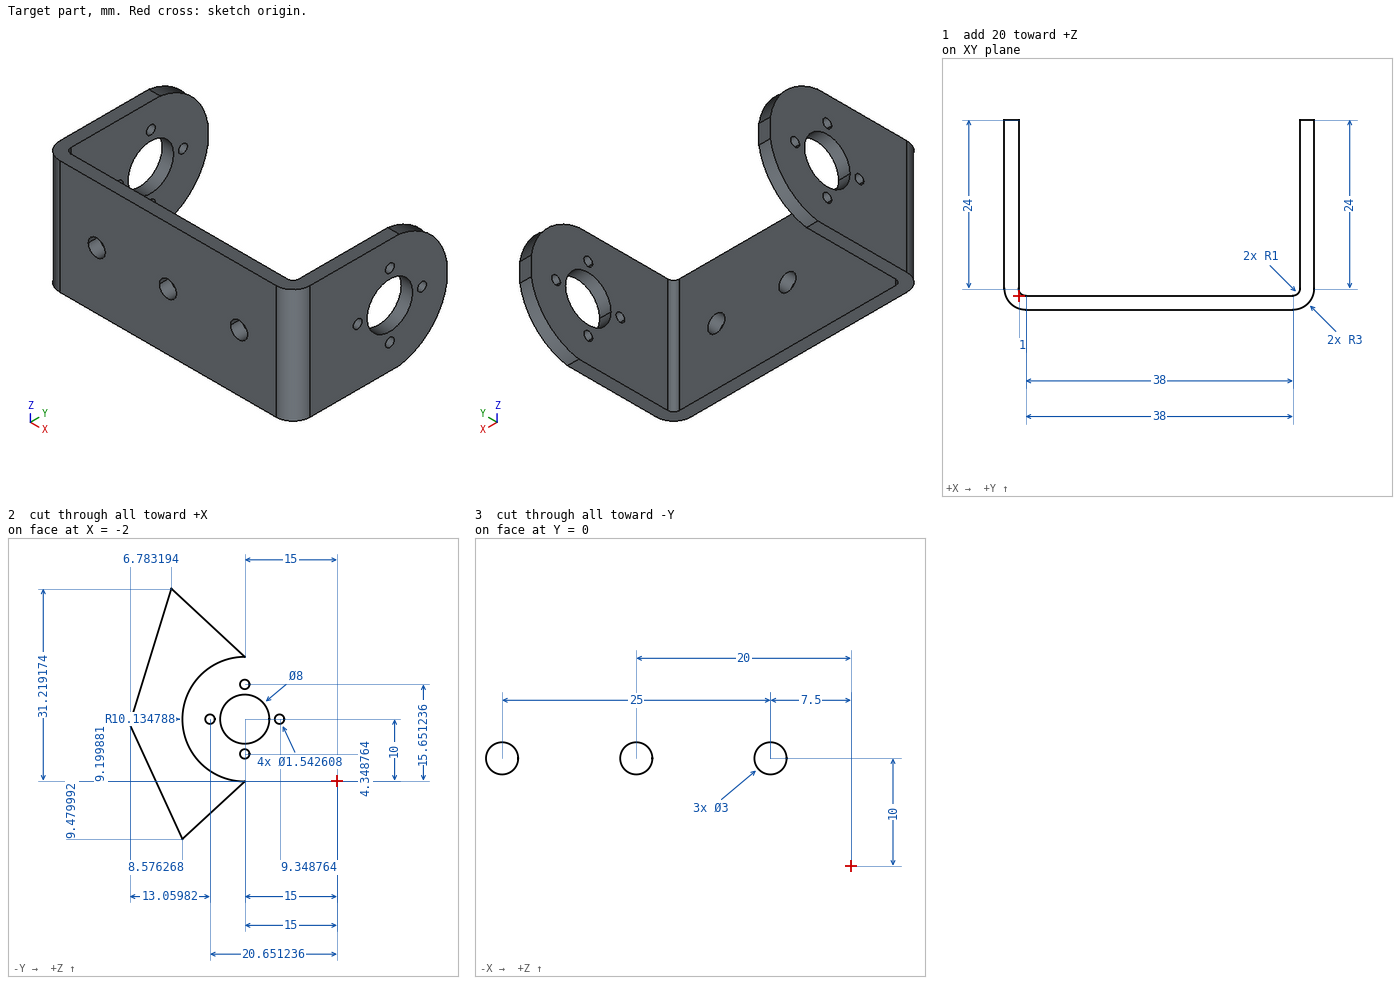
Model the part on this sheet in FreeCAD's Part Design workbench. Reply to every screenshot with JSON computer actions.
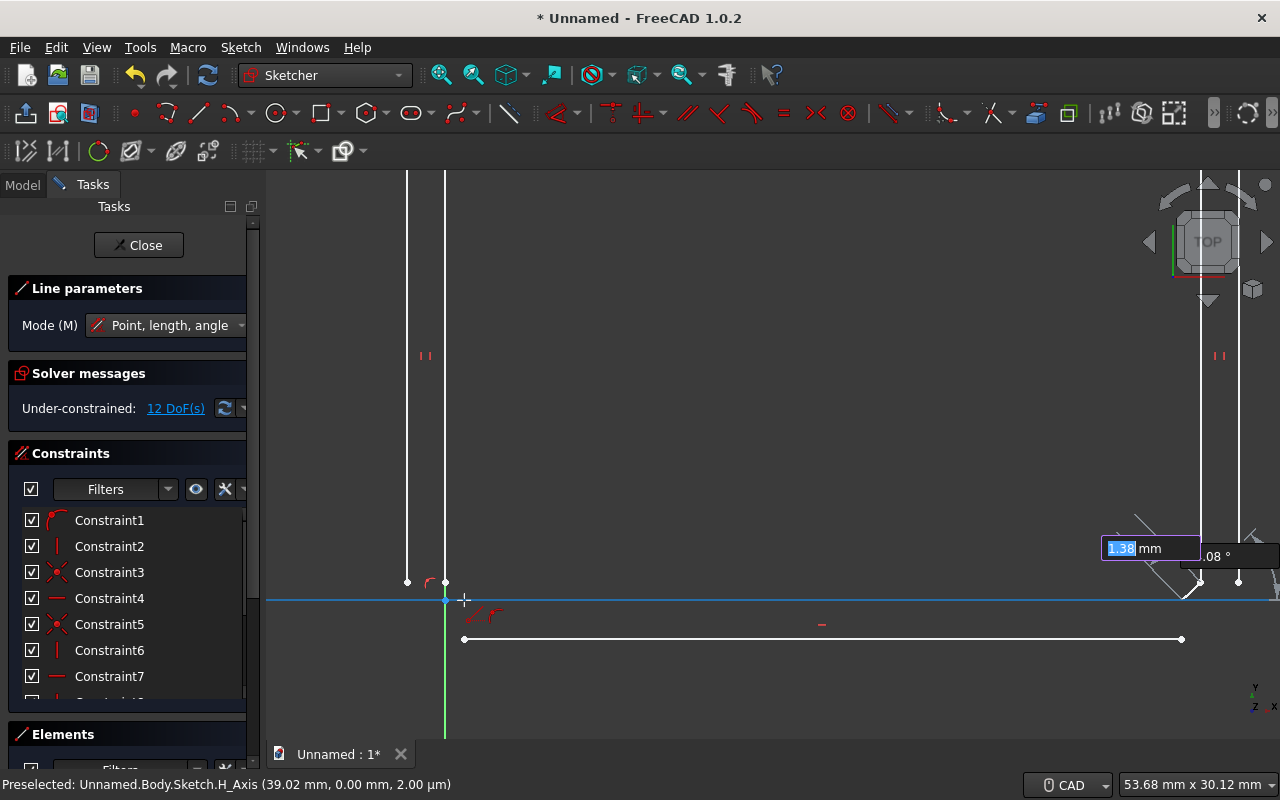
{"action": "left_click", "coordinate": [464, 591]}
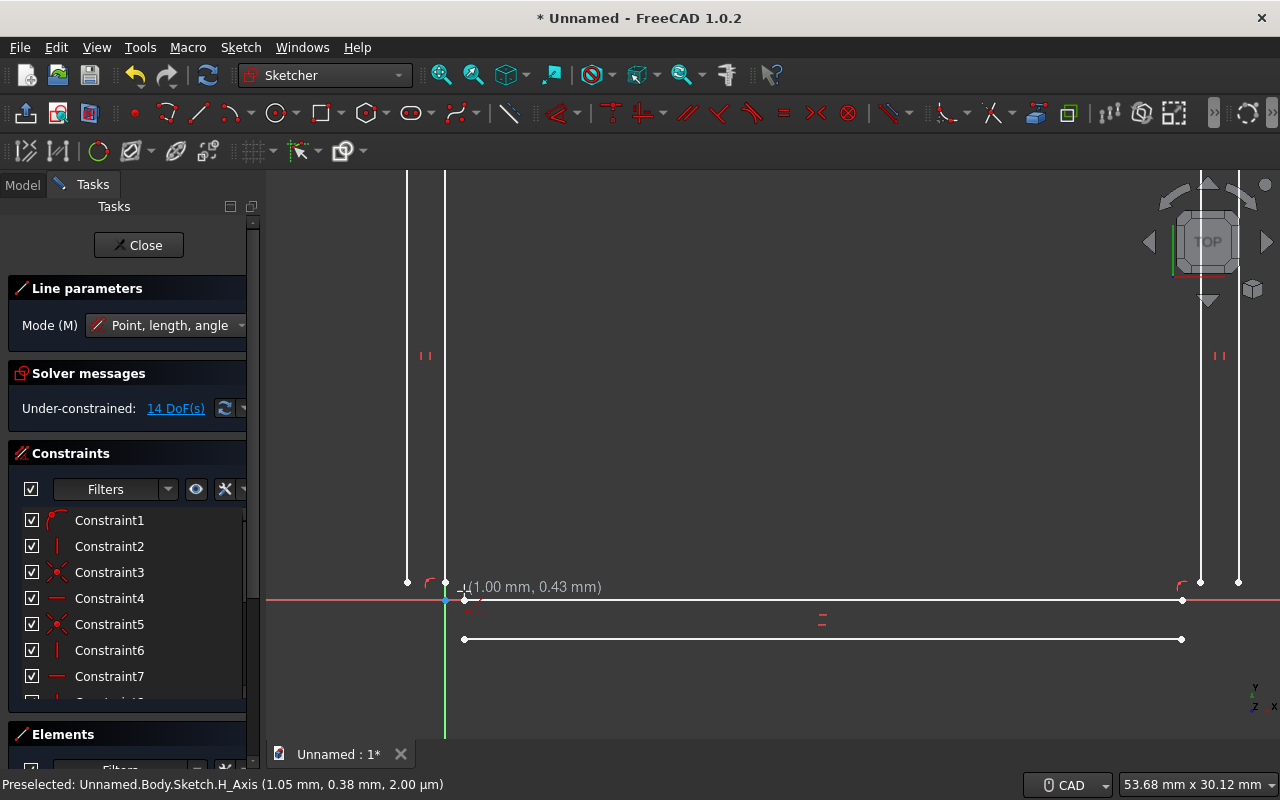
{"action": "left_click", "coordinate": [254, 114]}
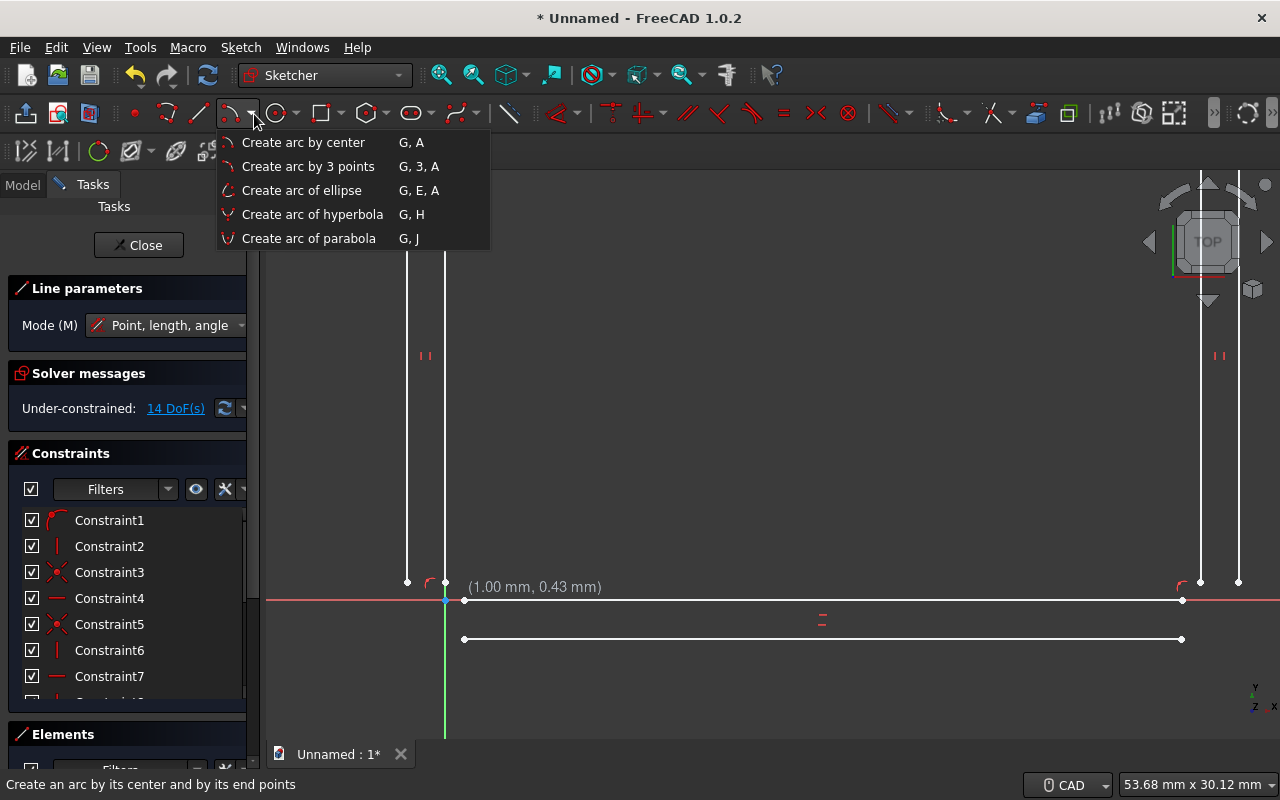
{"action": "left_click", "coordinate": [354, 166]}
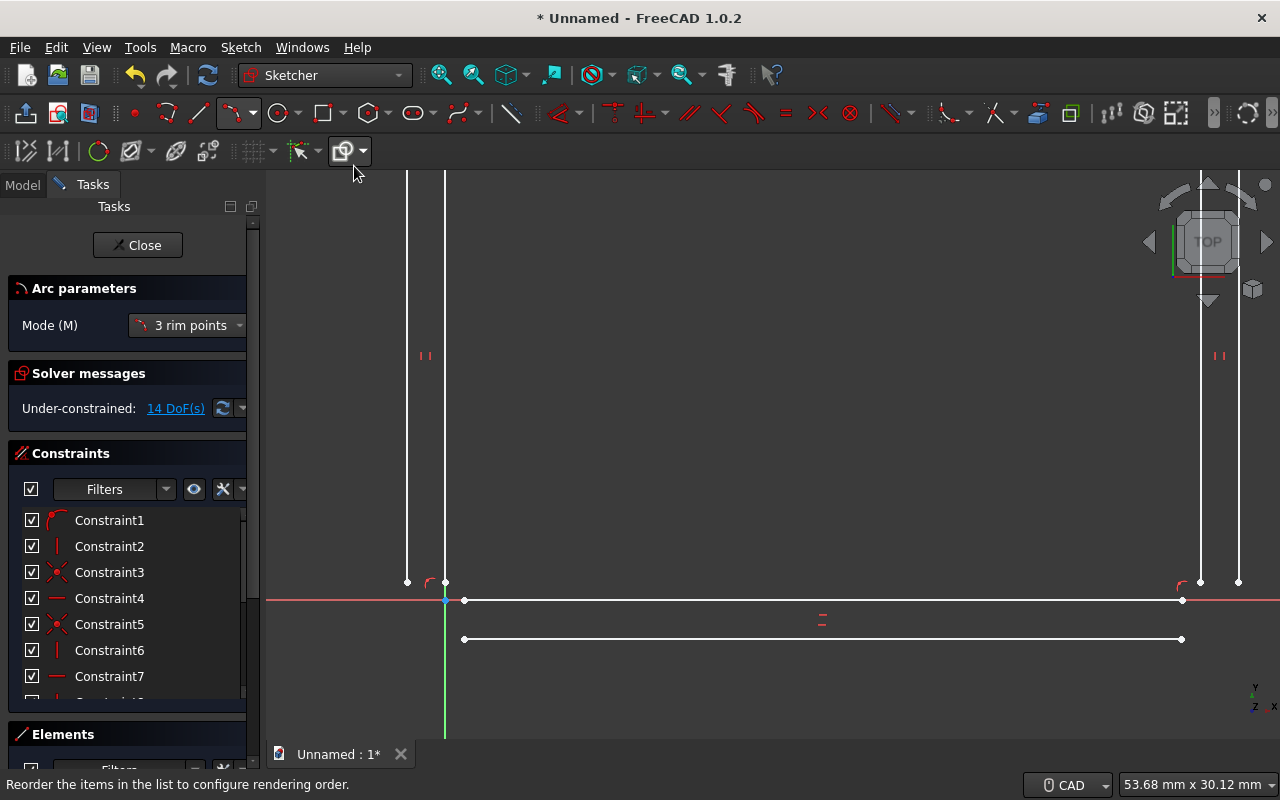
{"action": "left_click", "coordinate": [407, 582]}
{"action": "left_click", "coordinate": [464, 639]}
{"action": "left_click", "coordinate": [424, 621]}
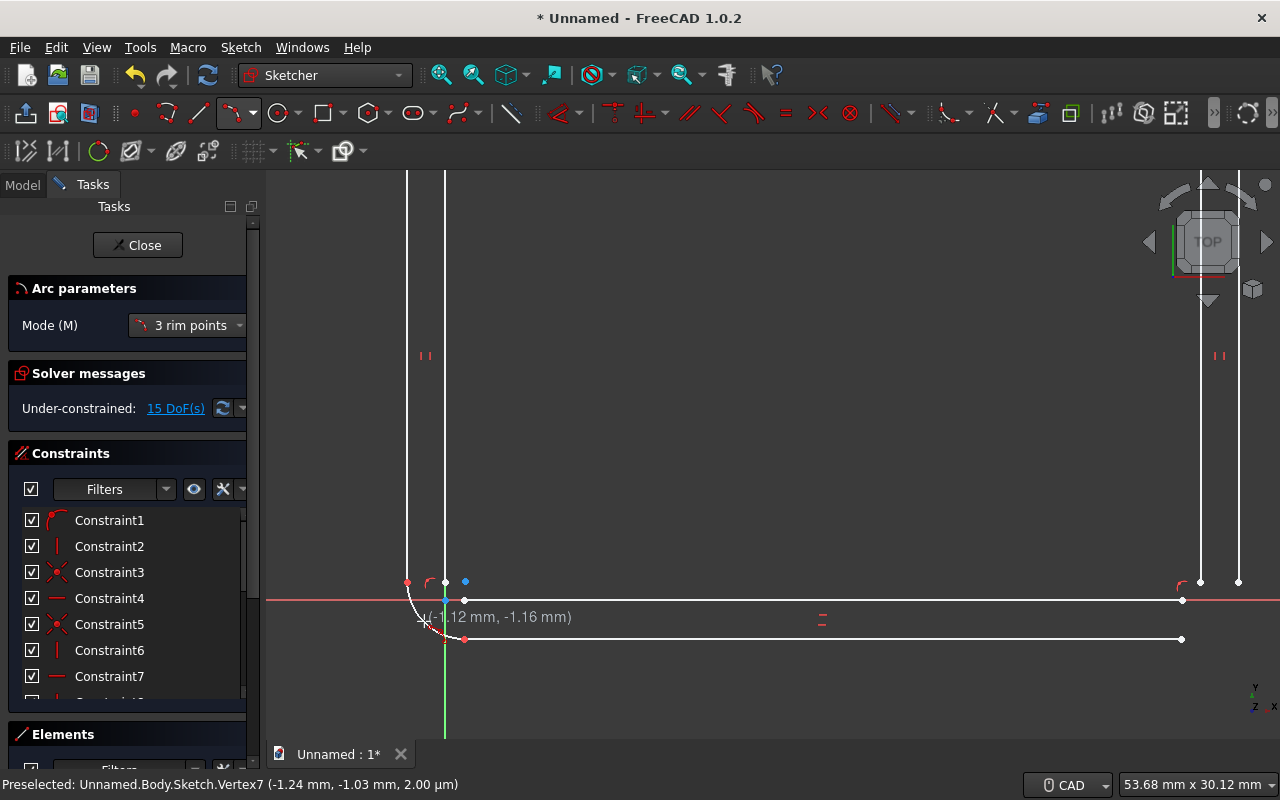
{"action": "scroll", "coordinate": [464, 600], "scroll_direction": "down", "scroll_amount": 2}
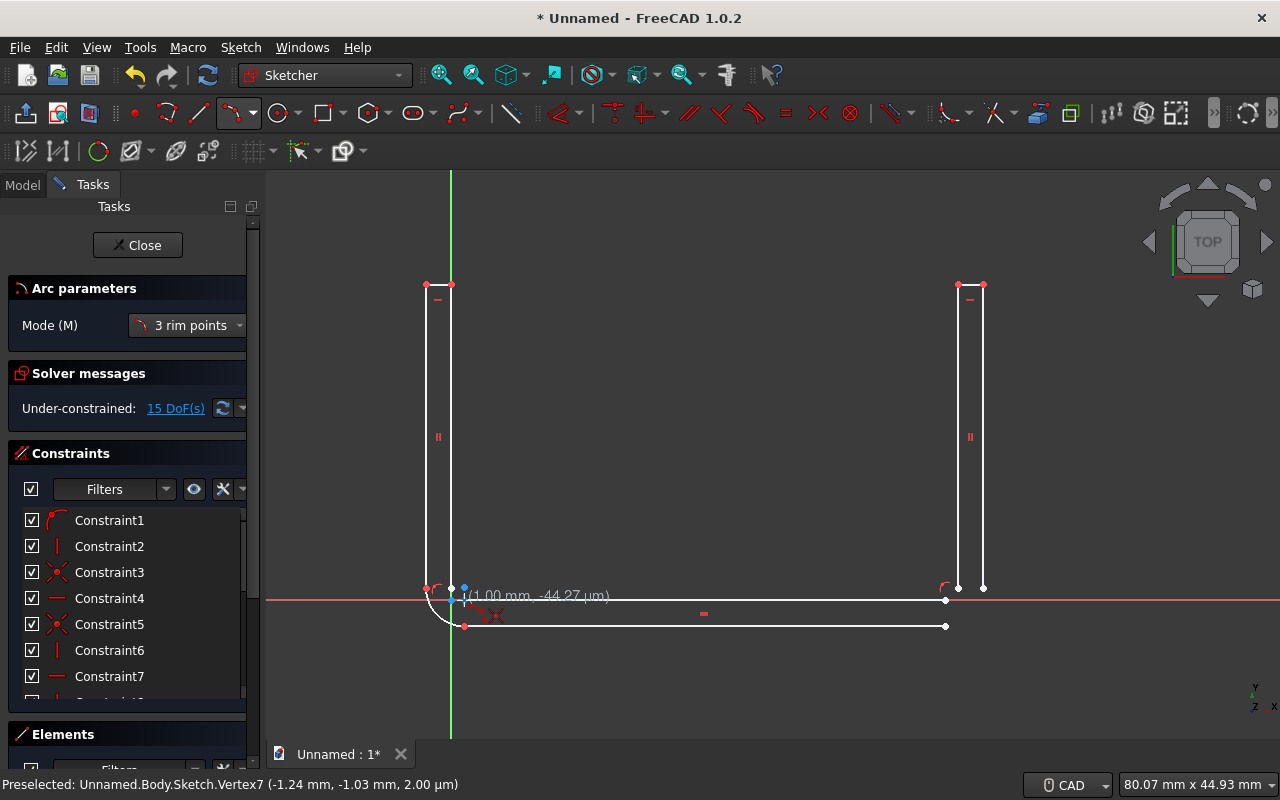
{"action": "left_click", "coordinate": [945, 626]}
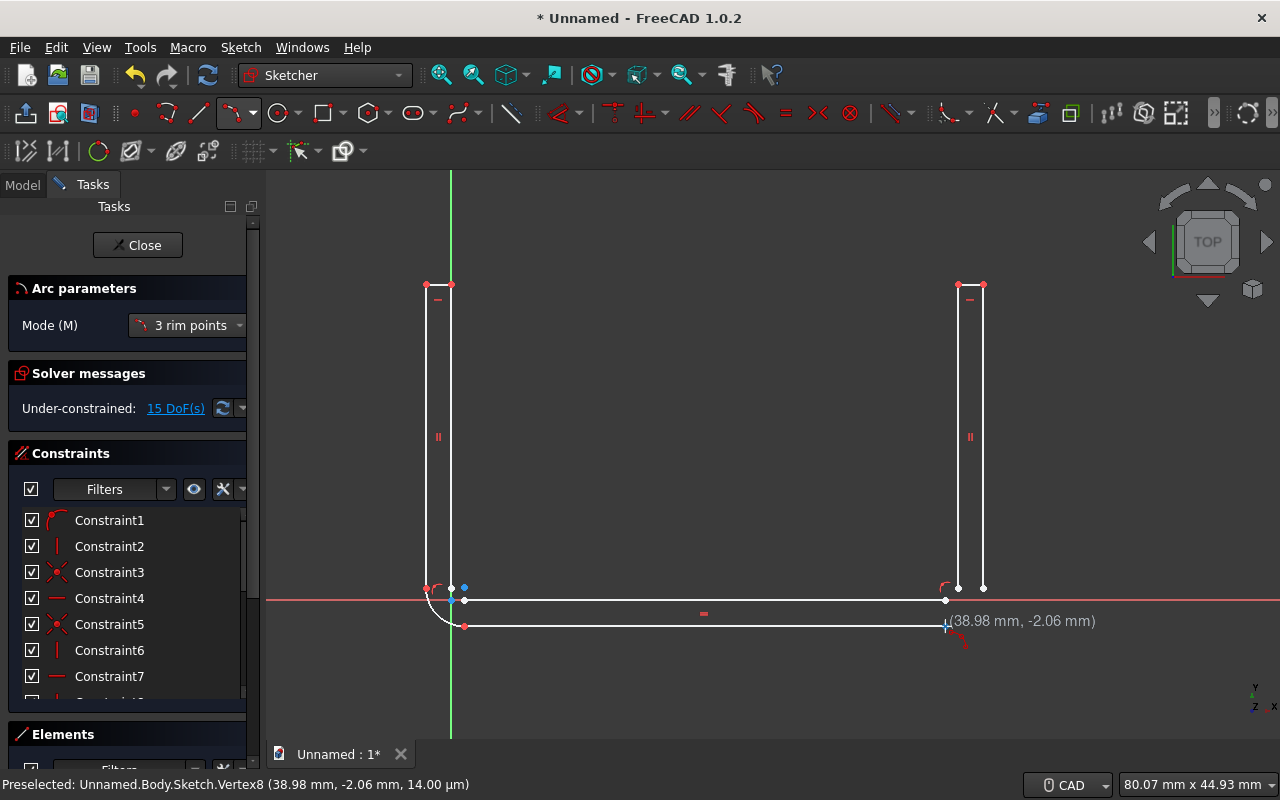
{"action": "scroll", "coordinate": [983, 588], "scroll_direction": "up", "scroll_amount": 2}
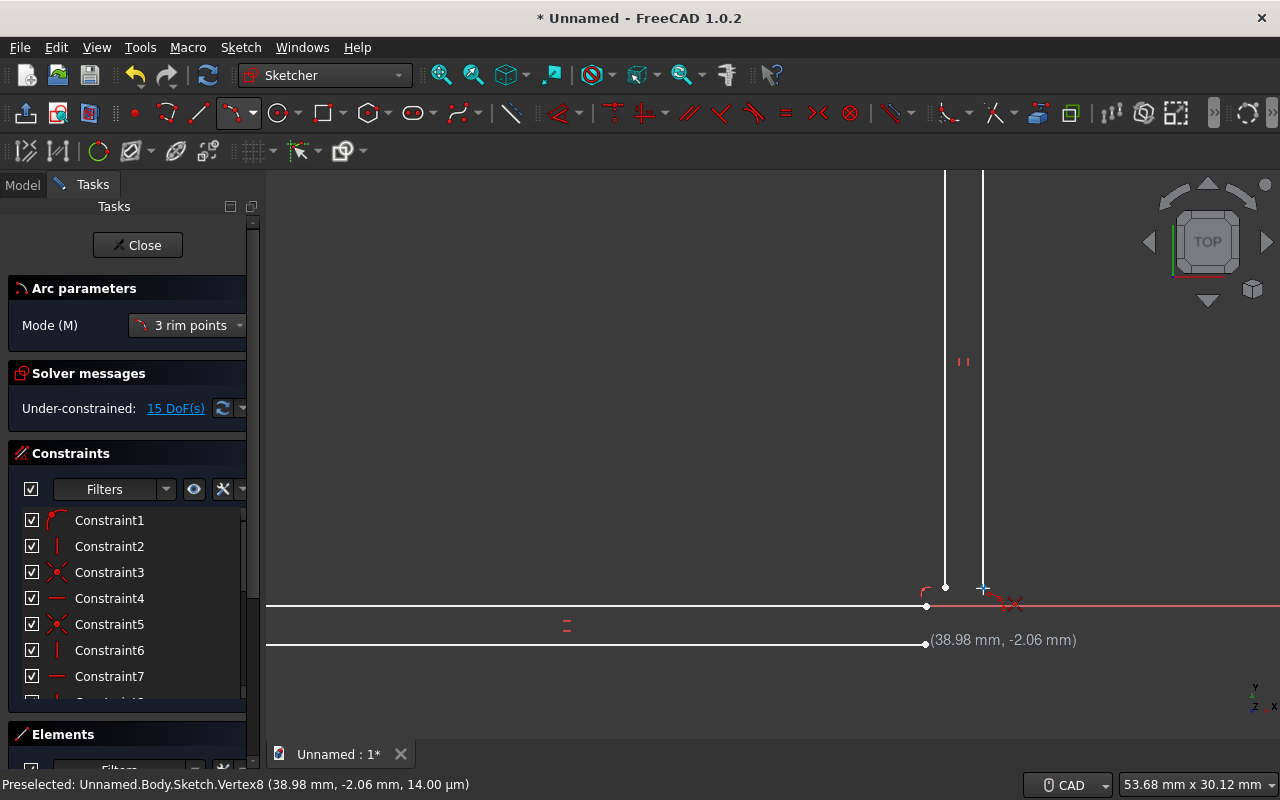
{"action": "left_click", "coordinate": [983, 588]}
{"action": "left_click", "coordinate": [966, 627]}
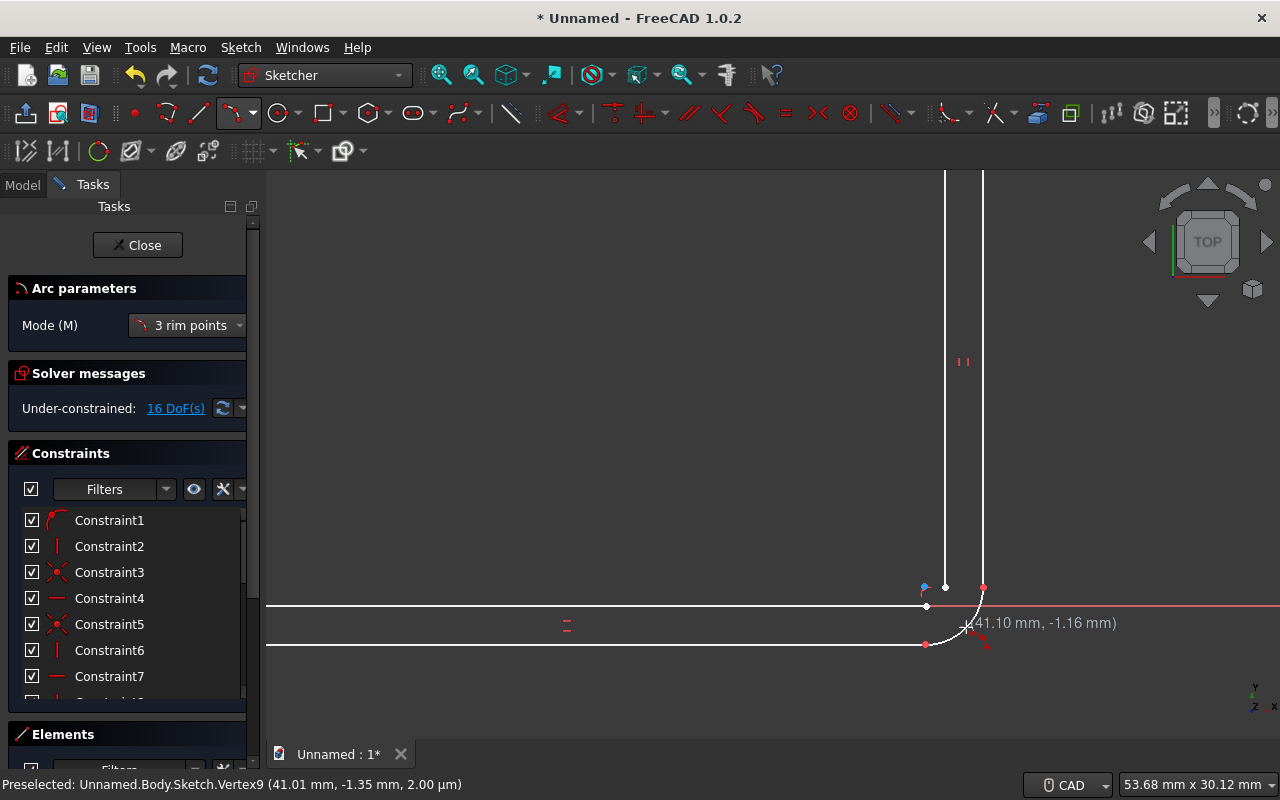
{"action": "left_click", "coordinate": [945, 588]}
{"action": "left_click", "coordinate": [927, 606]}